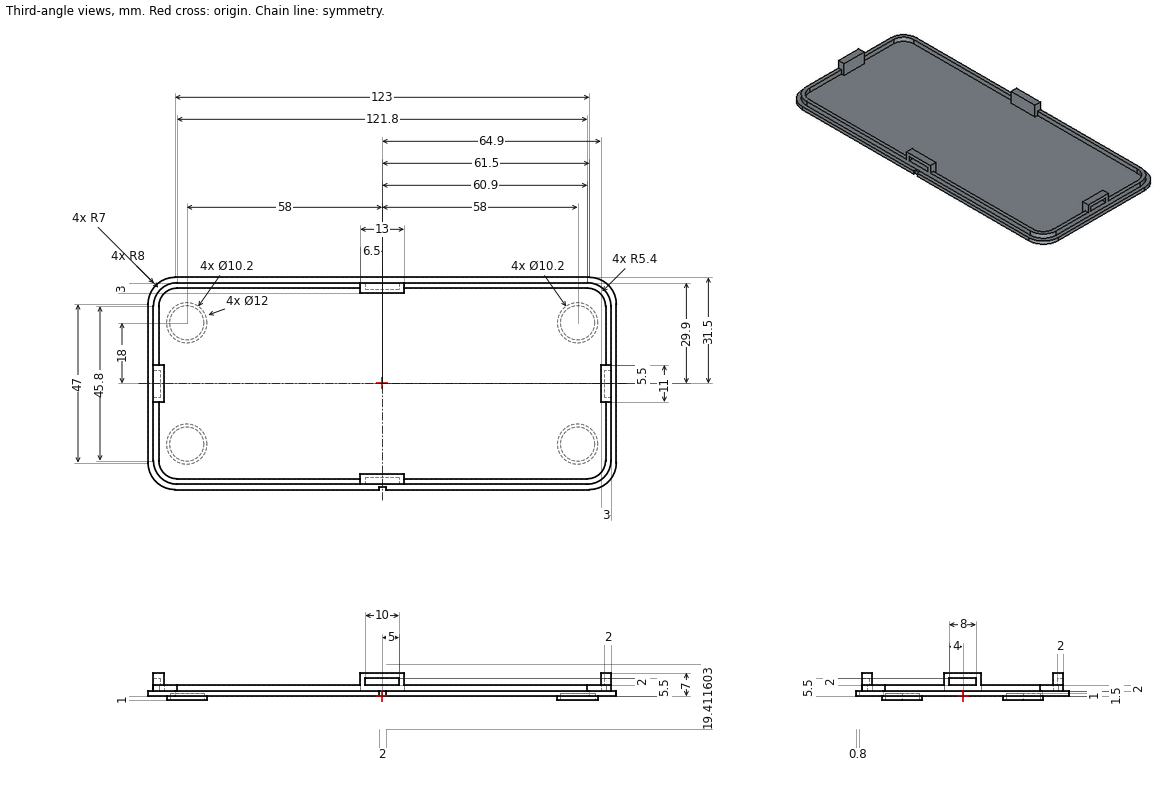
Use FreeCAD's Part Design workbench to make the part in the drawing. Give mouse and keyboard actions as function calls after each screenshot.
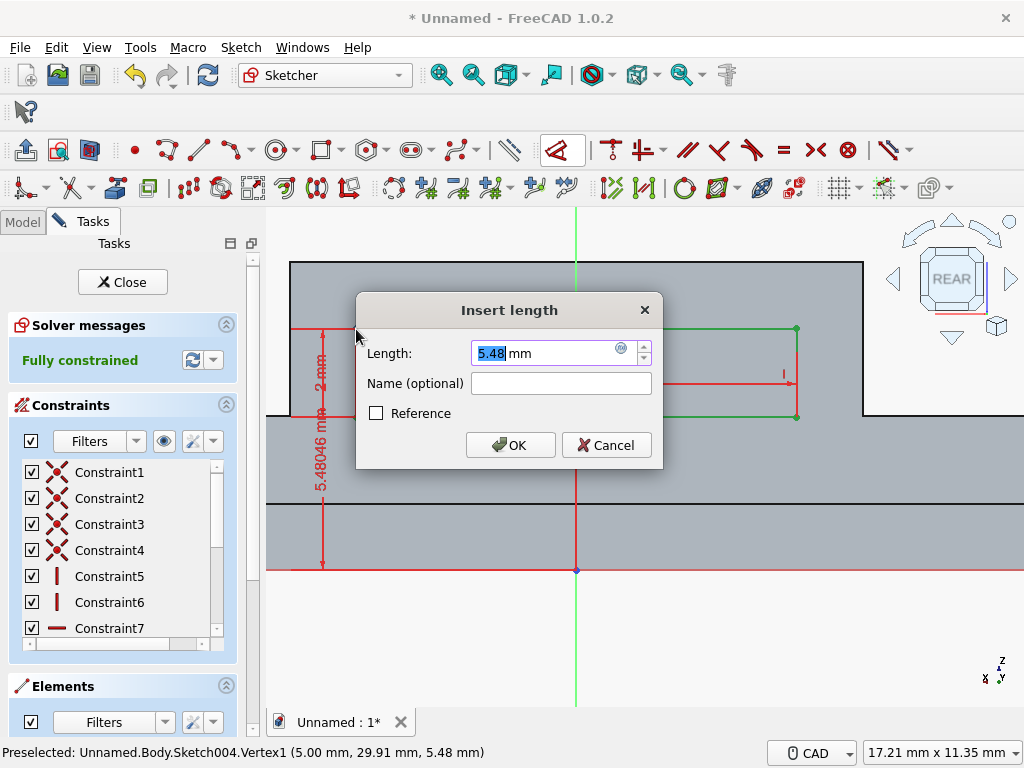
text(5.5)
key(Return)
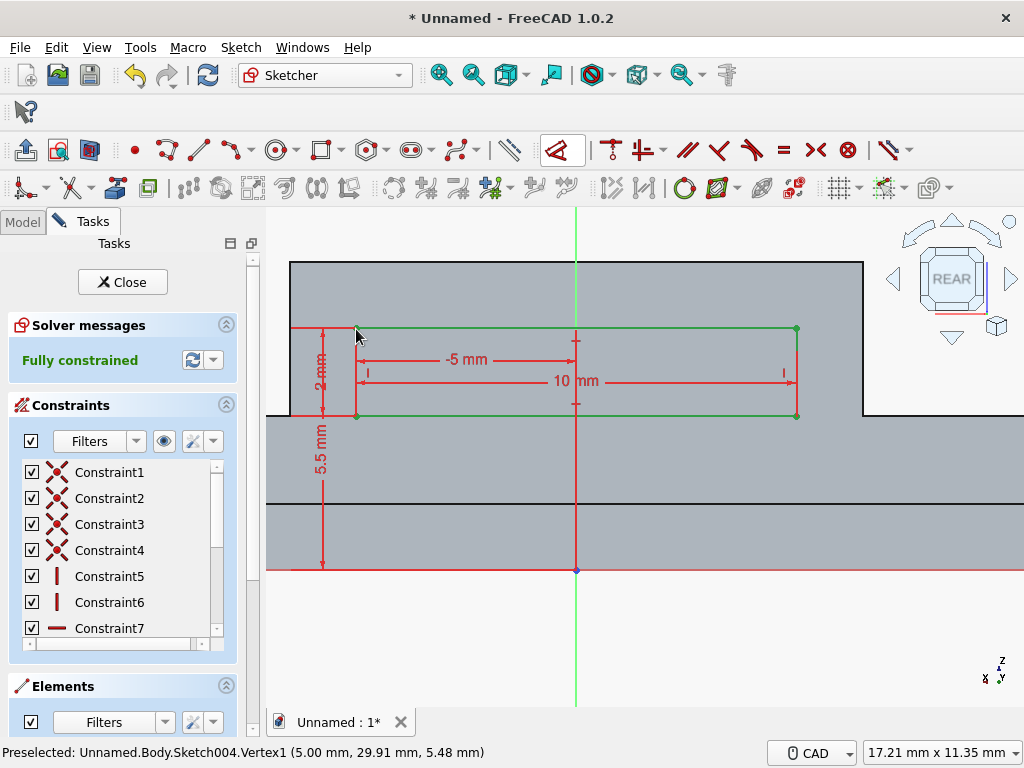
click(123, 282)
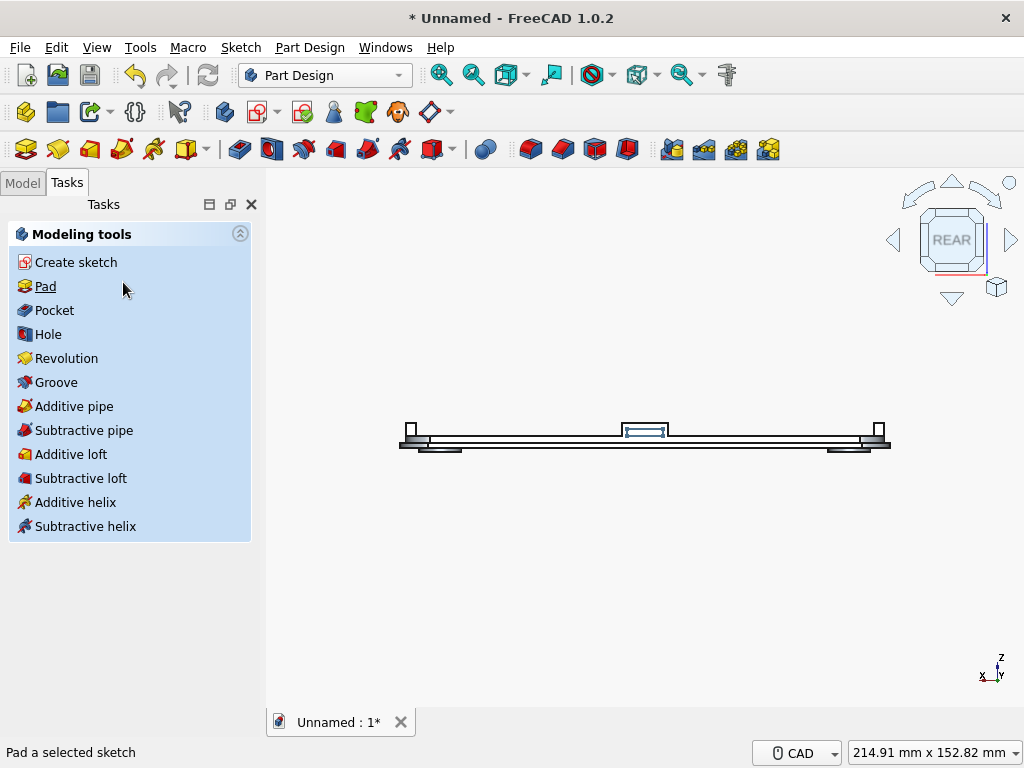
click(240, 150)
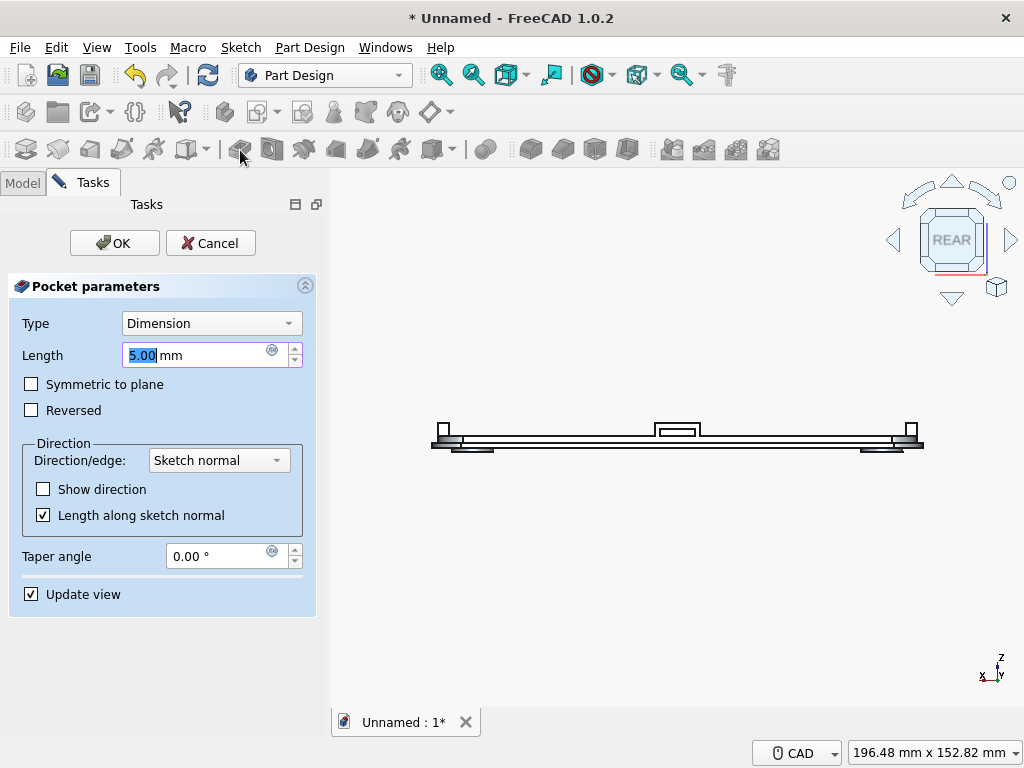
text(2)
key(Tab)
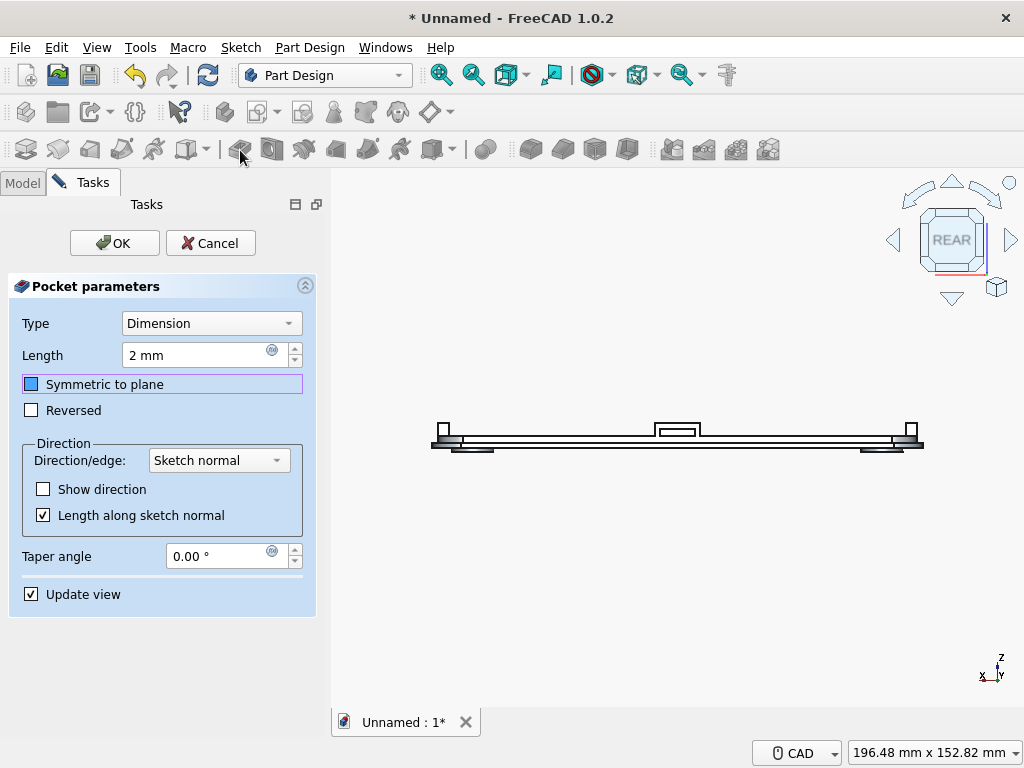
click(115, 243)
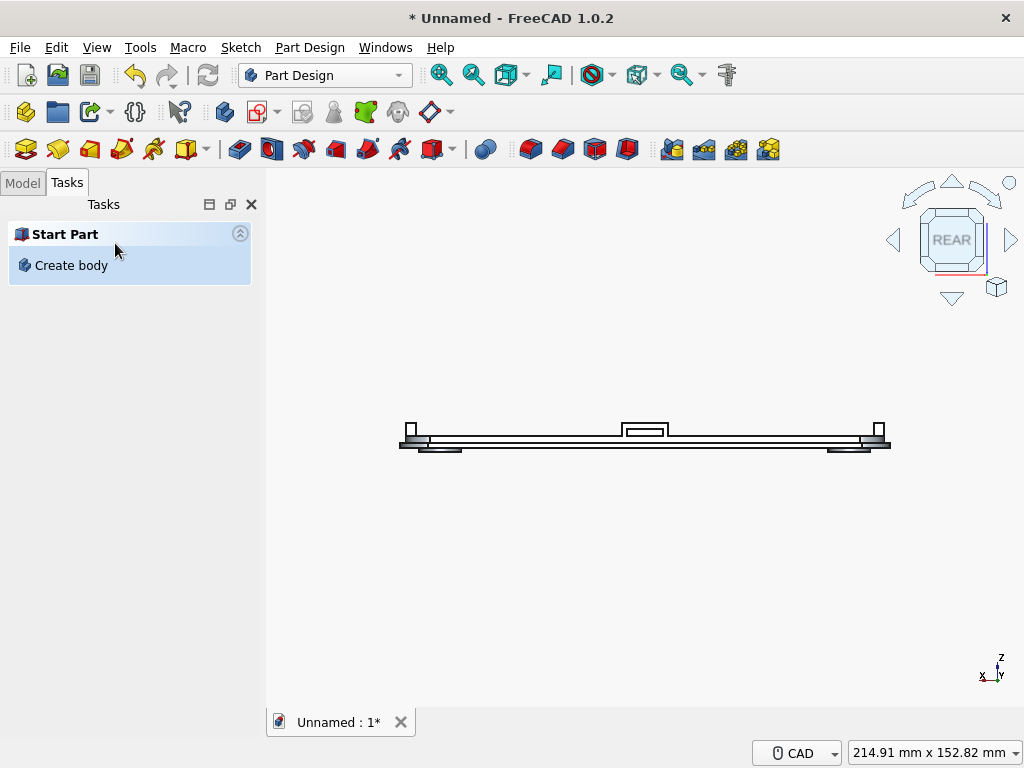
click(23, 182)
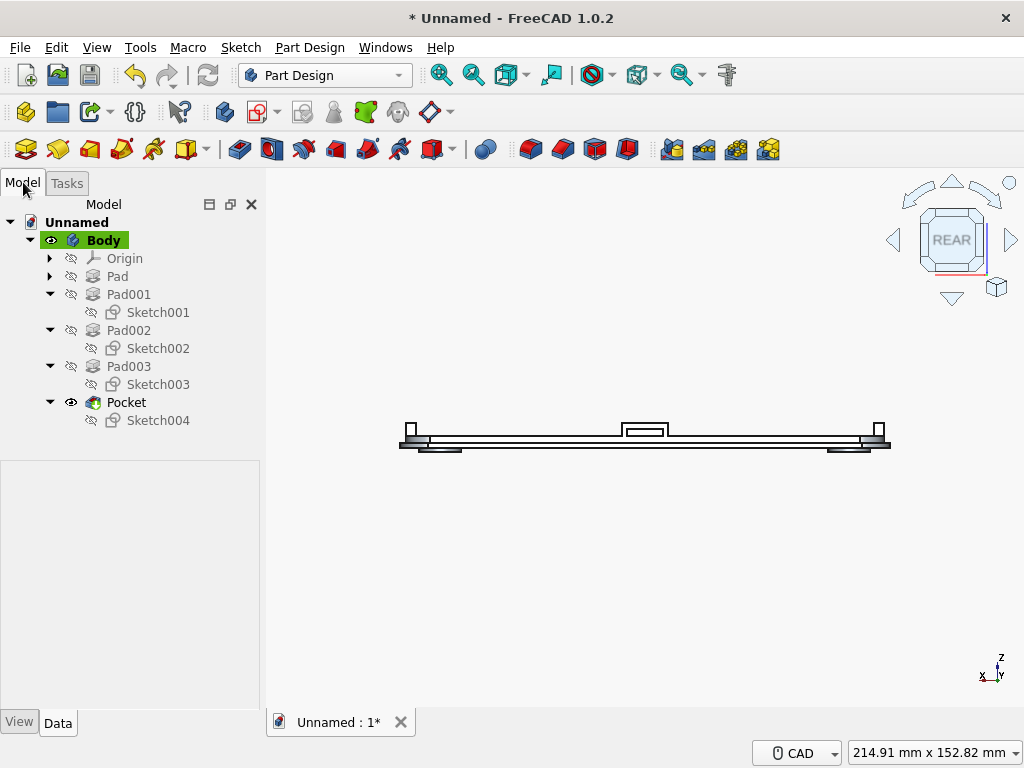
click(116, 402)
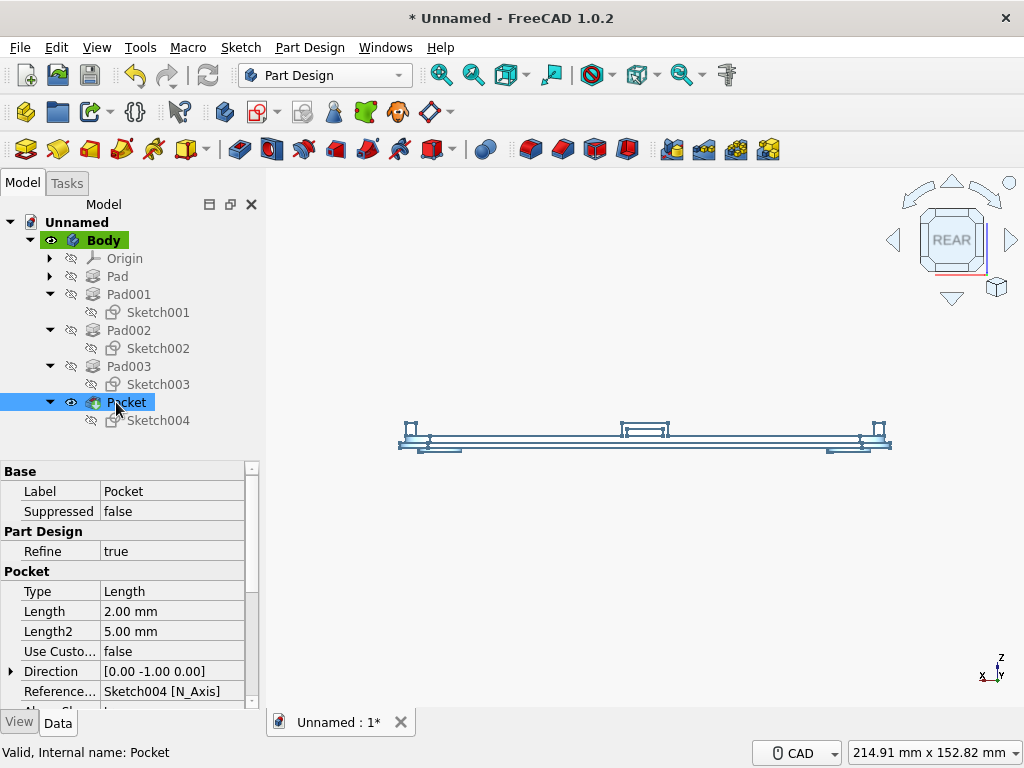
click(672, 150)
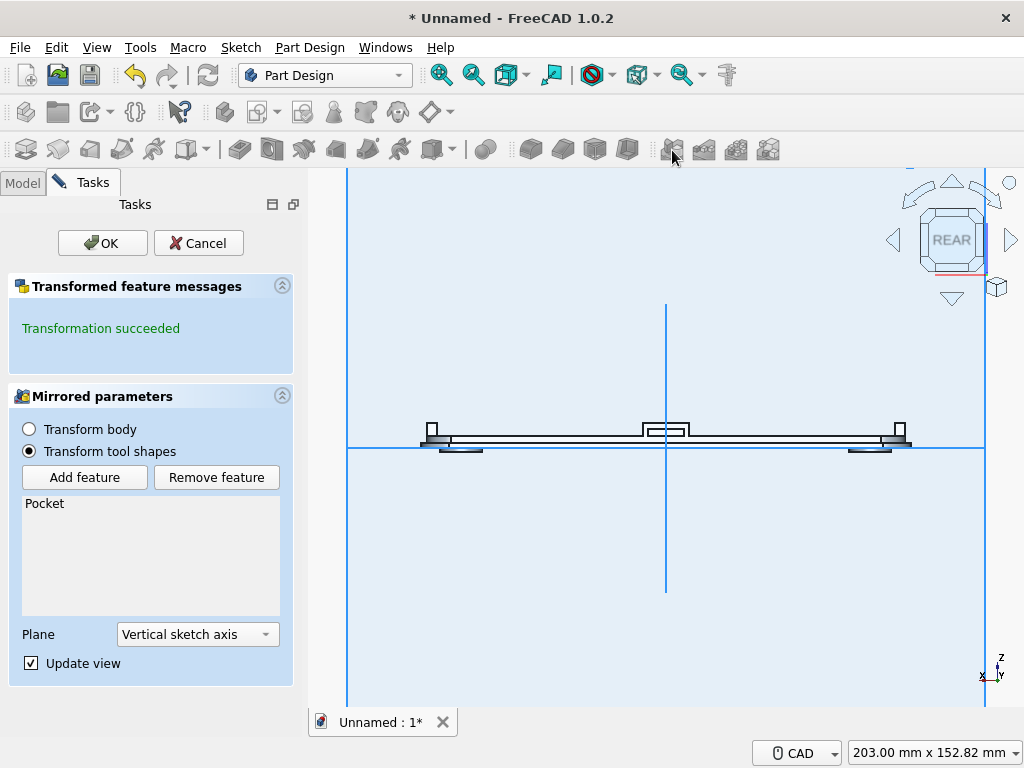
click(198, 634)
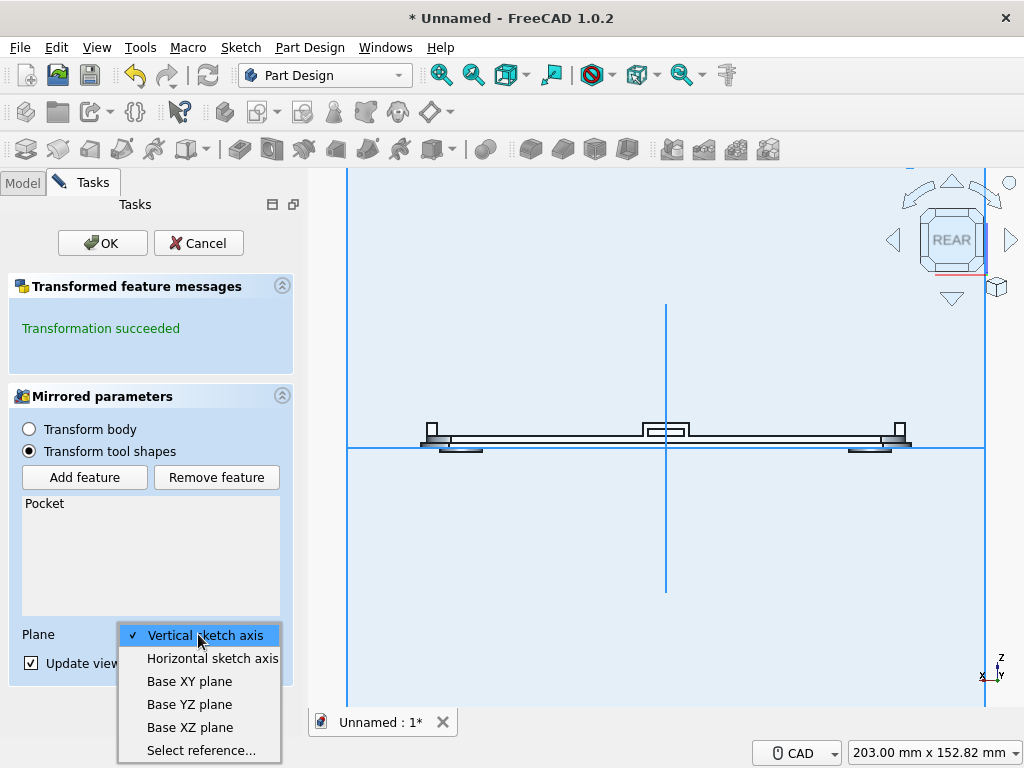
click(198, 728)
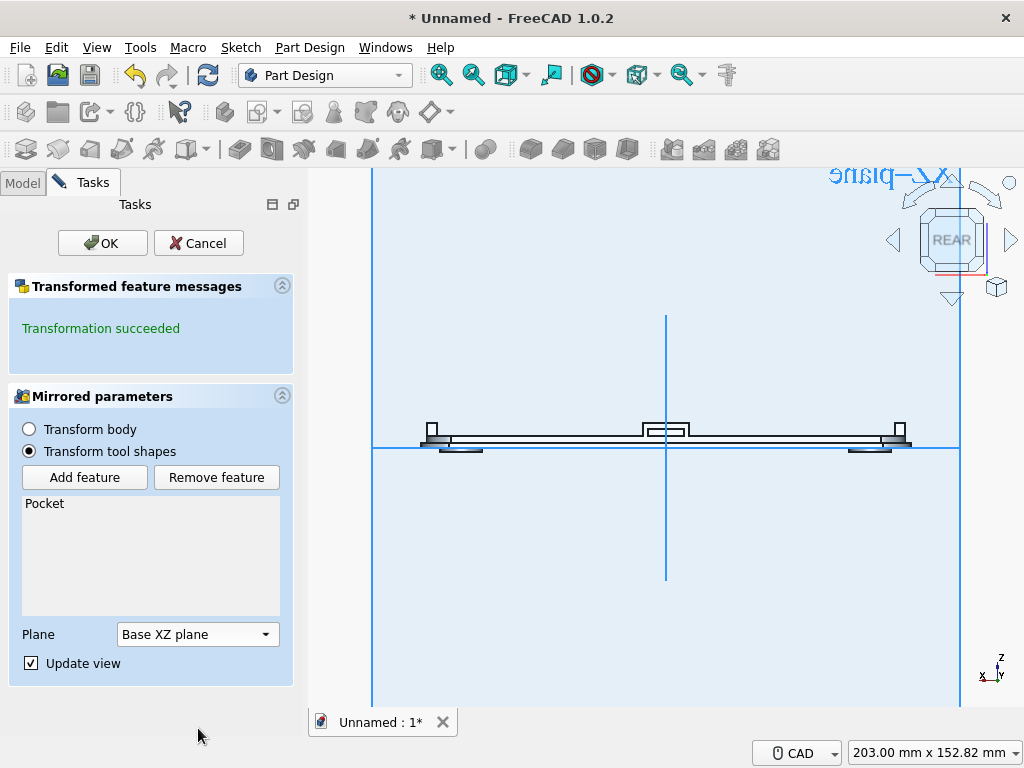
click(103, 243)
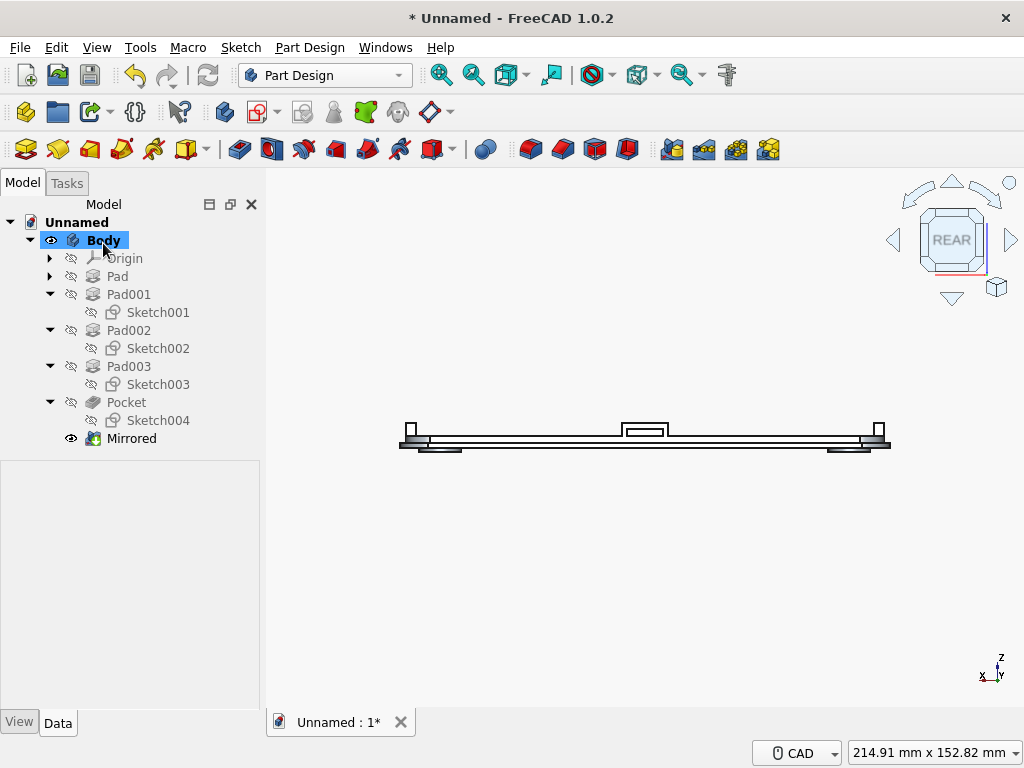
key(0)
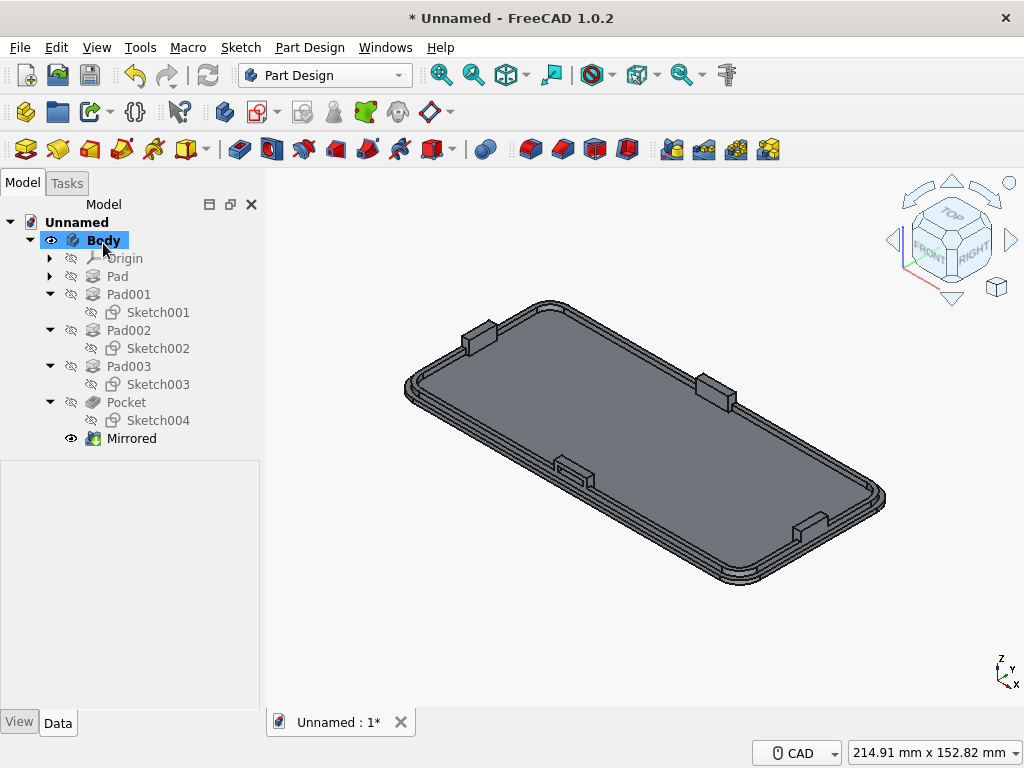
scroll(698, 564, up, 8)